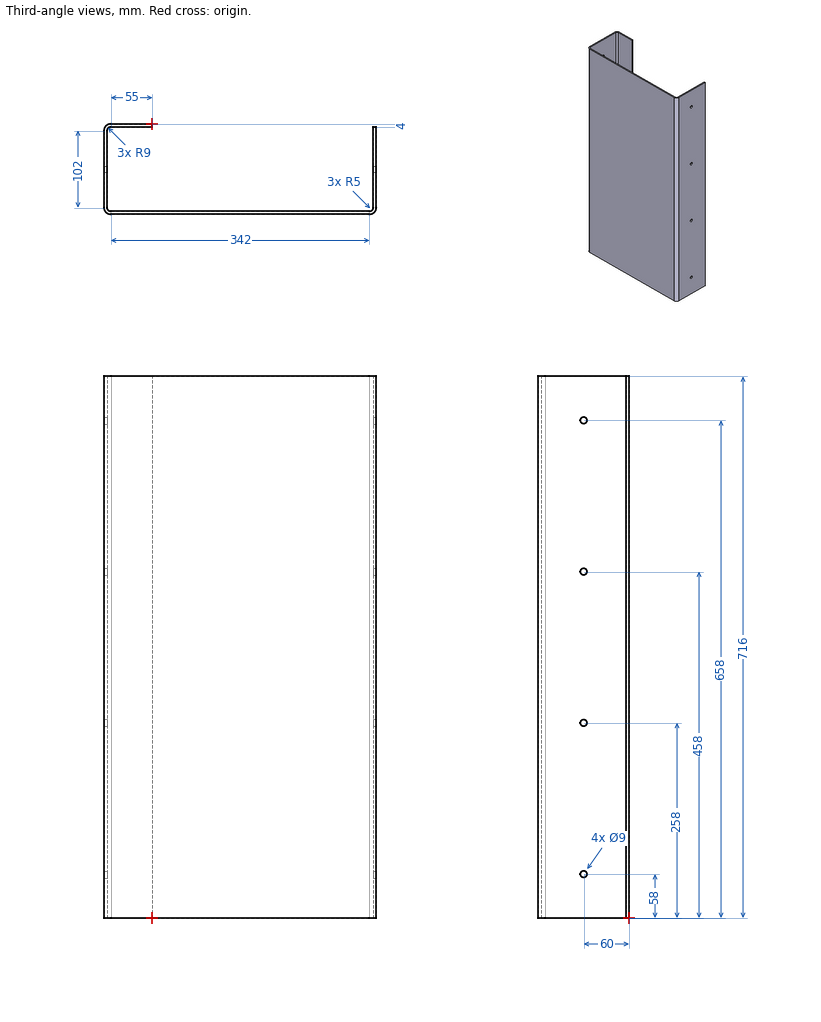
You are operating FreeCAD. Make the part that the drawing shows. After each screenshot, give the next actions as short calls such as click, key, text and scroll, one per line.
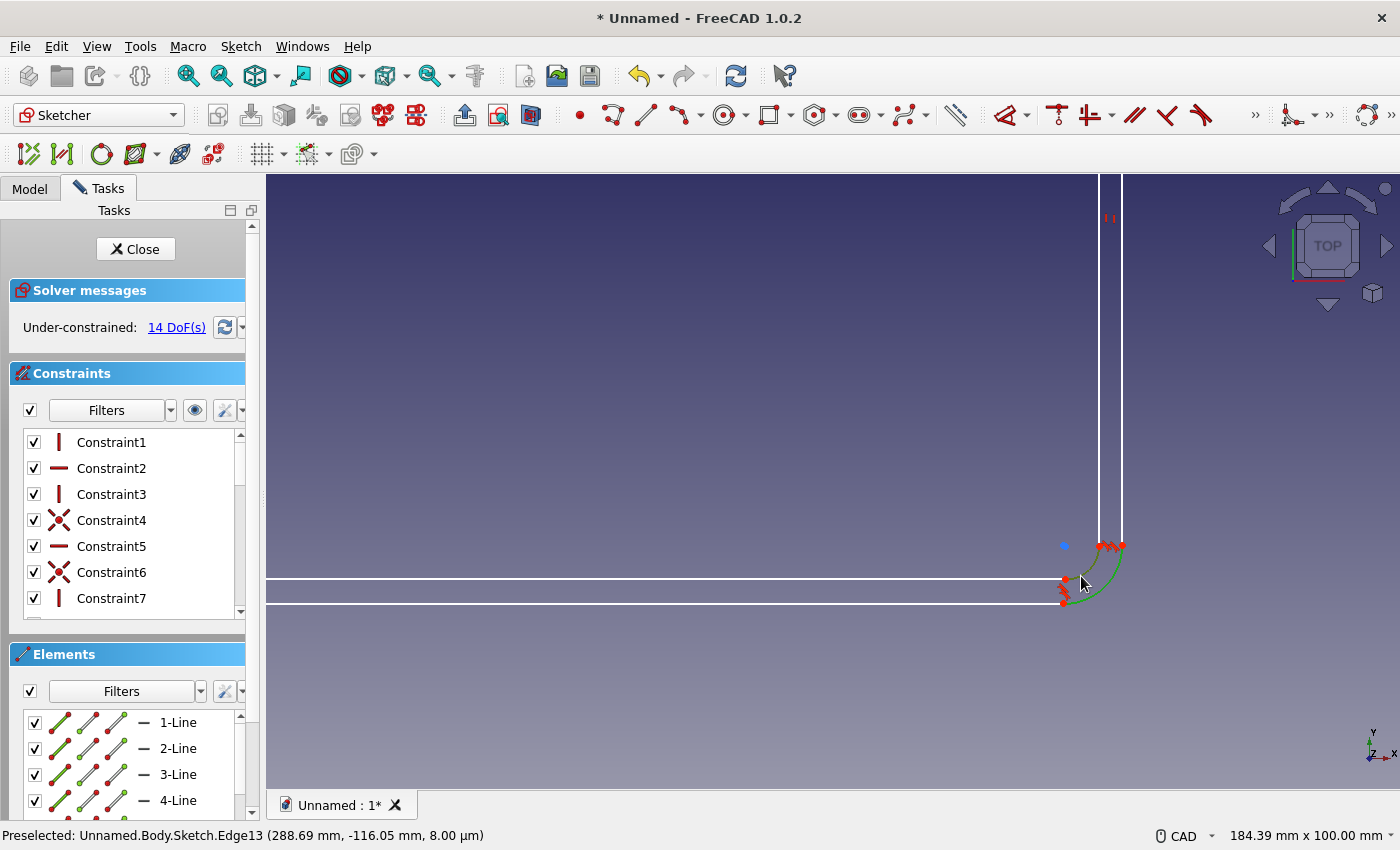
click(1057, 116)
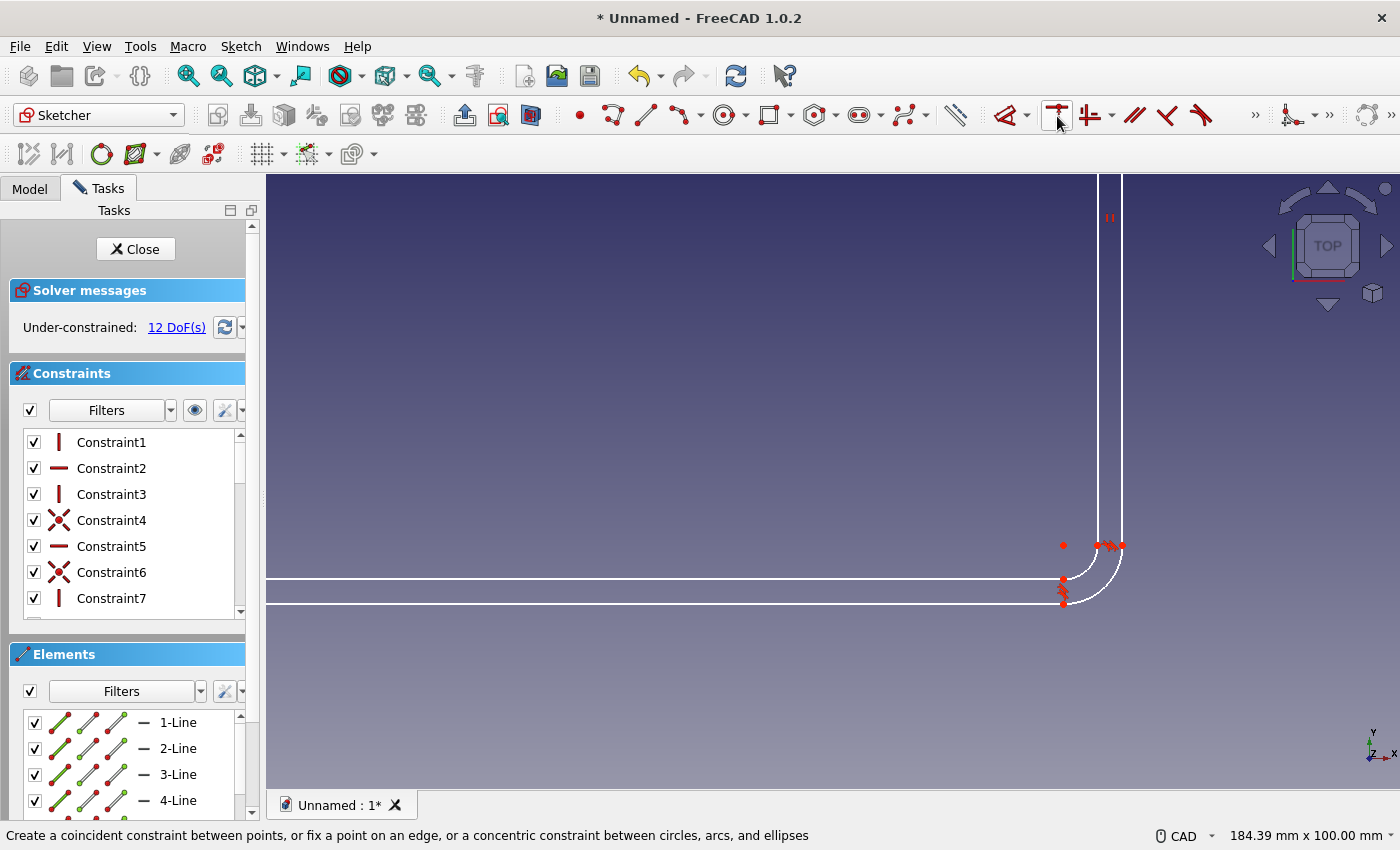
scroll(1088, 589, down, 6)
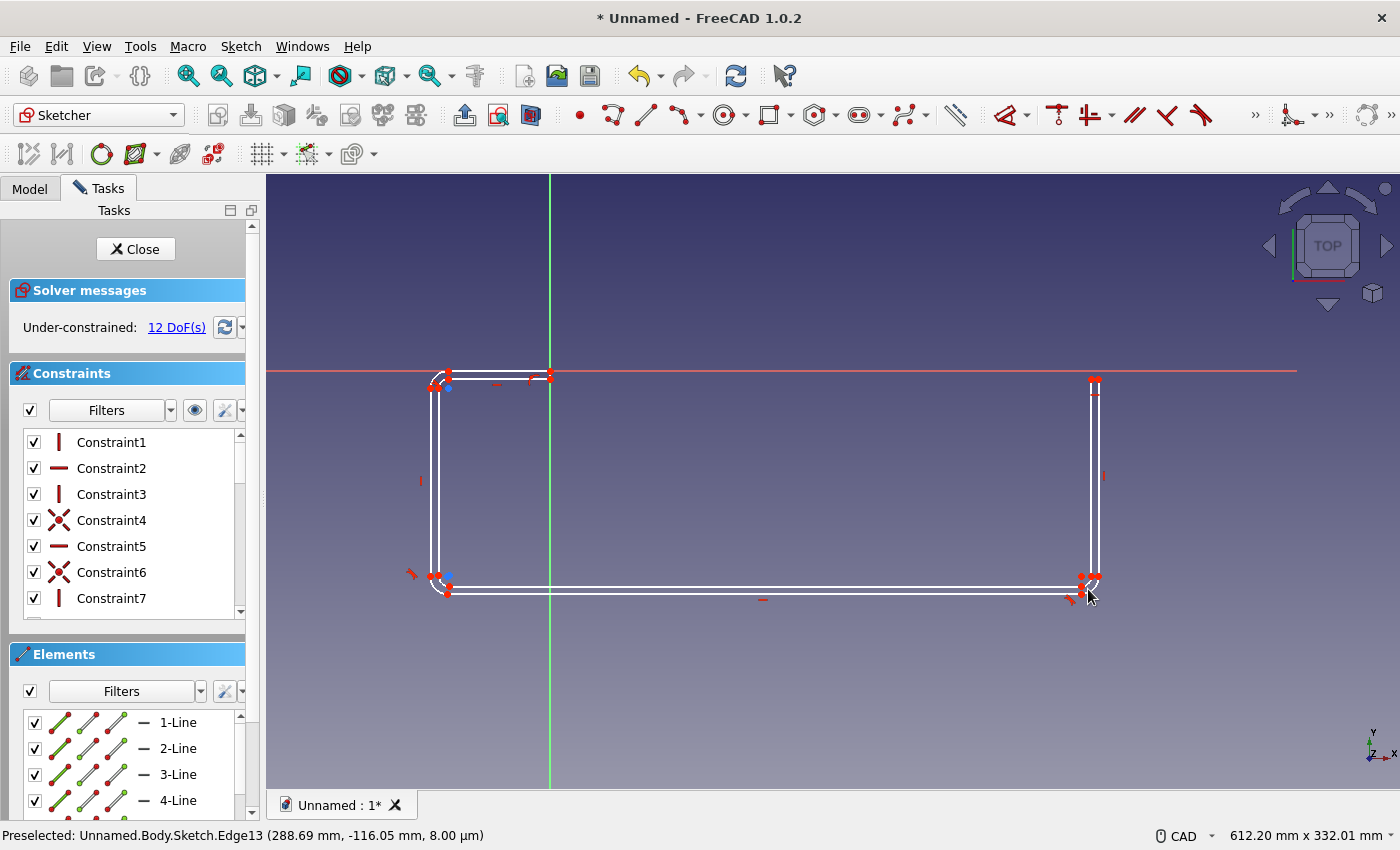
scroll(432, 585, up, 3)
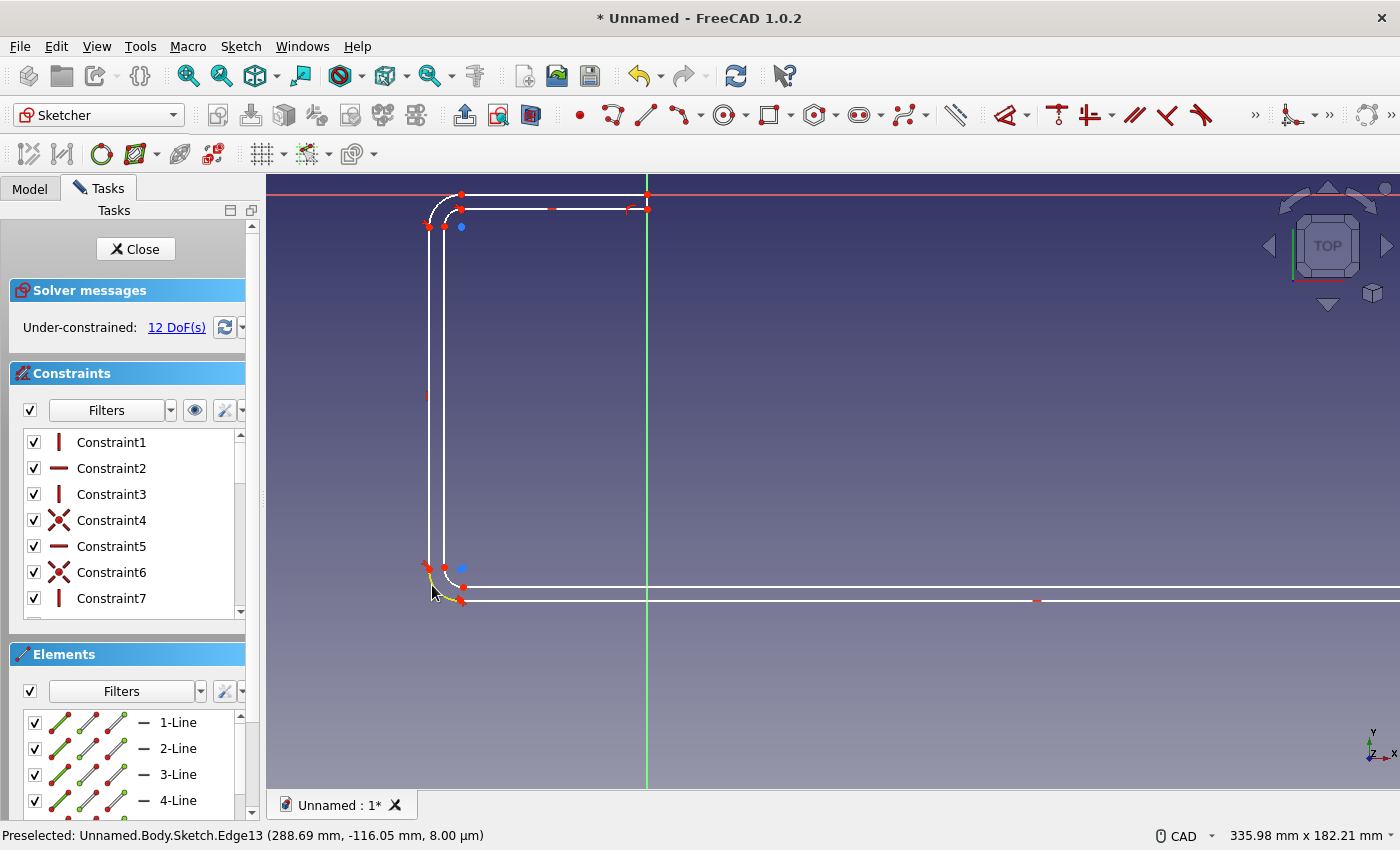
click(433, 584)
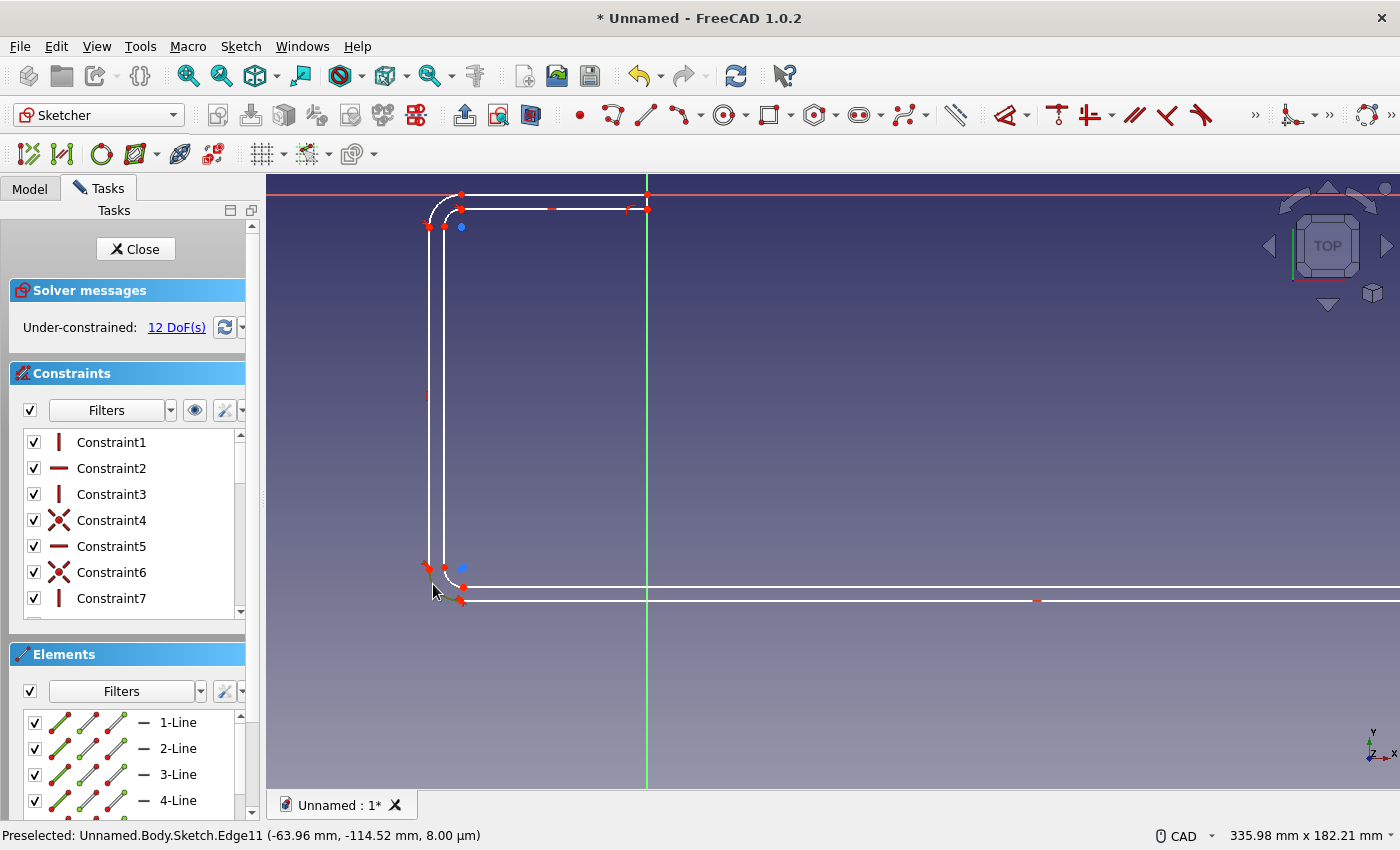
scroll(447, 577, up, 3)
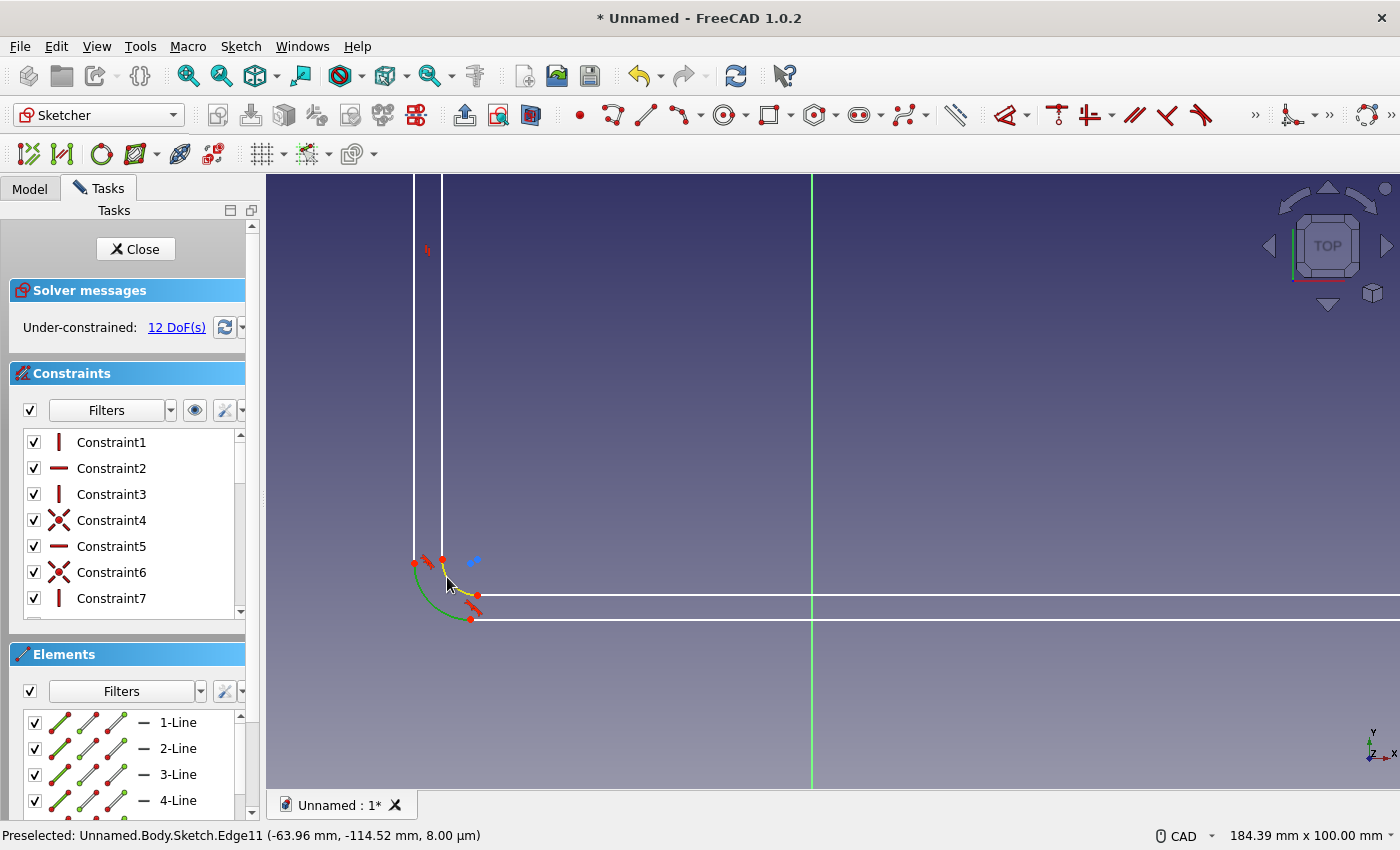
click(446, 576)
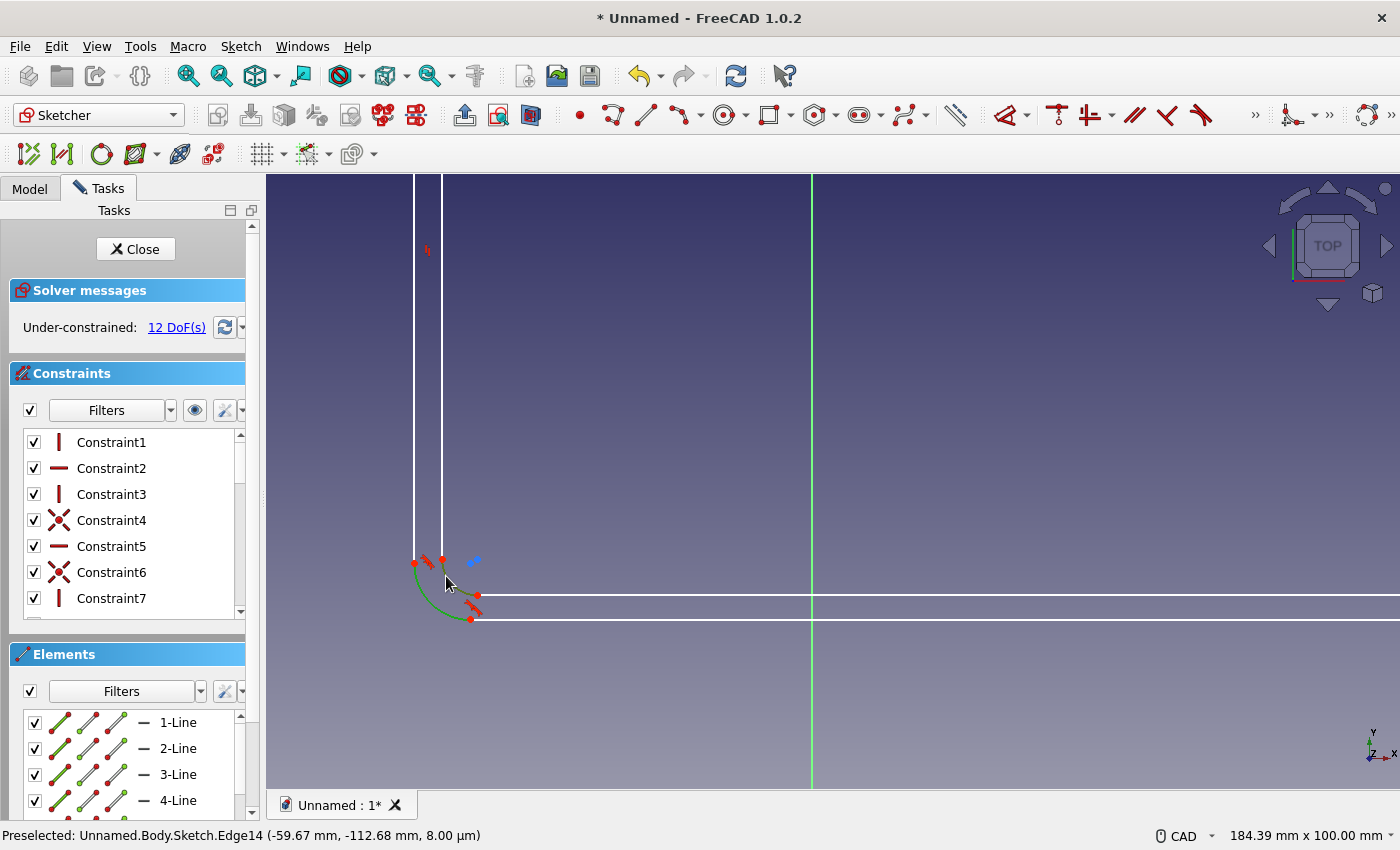
click(1057, 116)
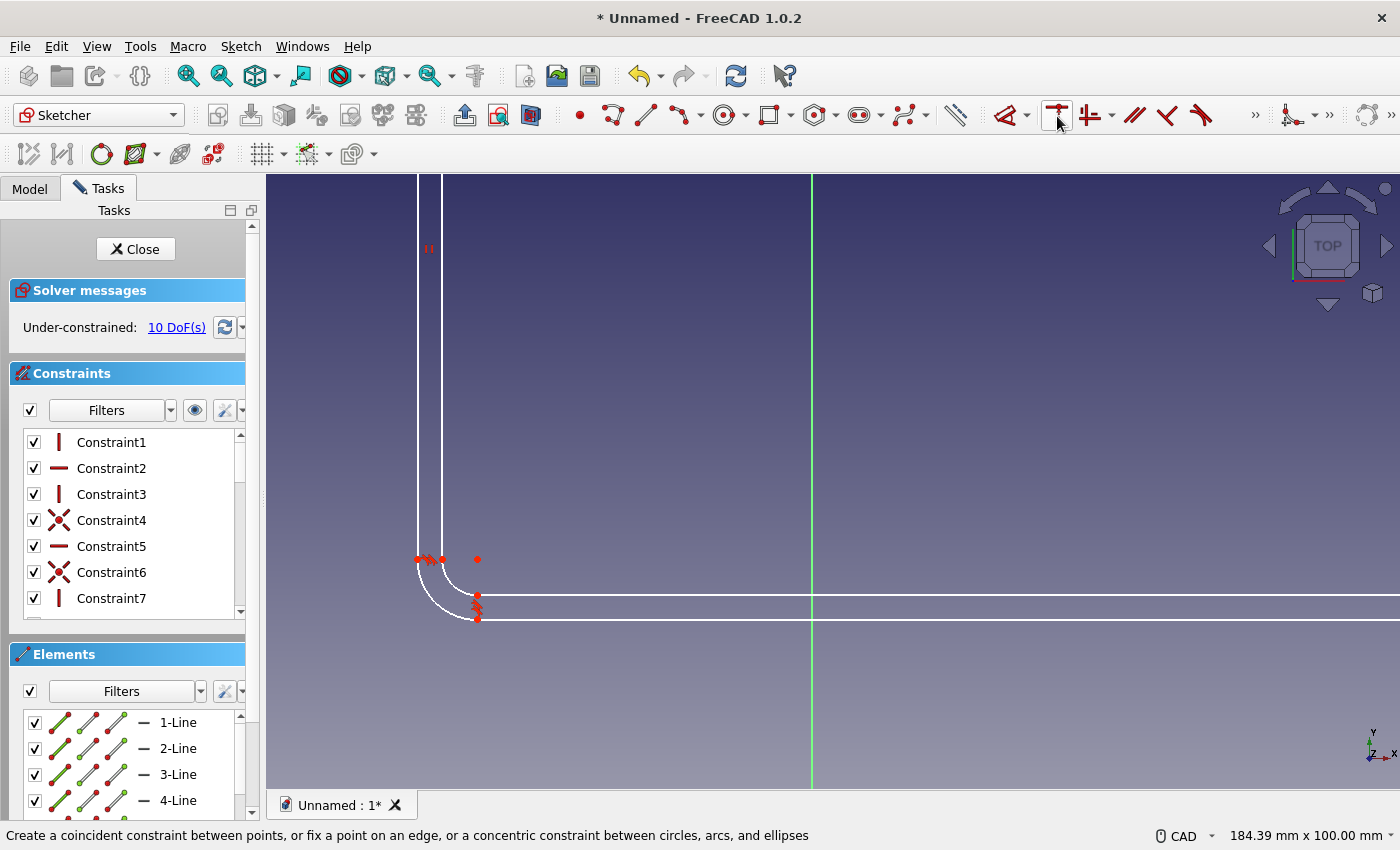
scroll(437, 582, down, 6)